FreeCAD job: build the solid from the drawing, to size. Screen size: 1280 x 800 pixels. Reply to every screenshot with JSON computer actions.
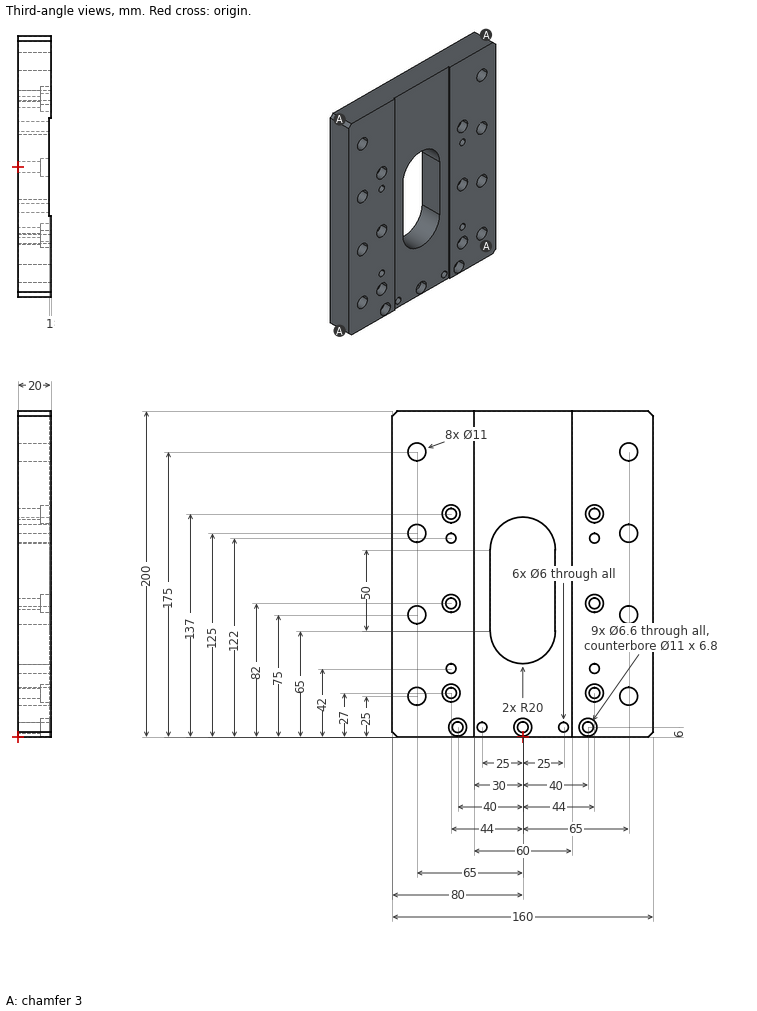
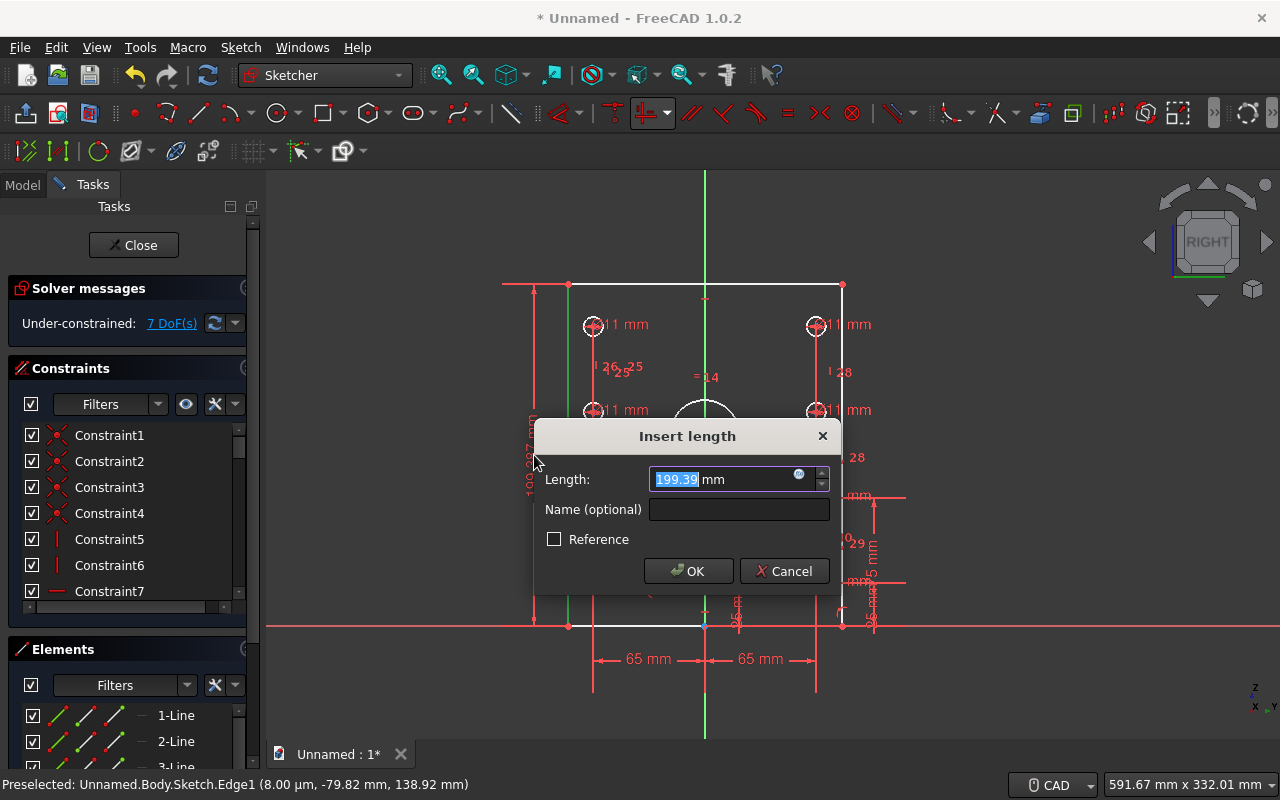
{"action": "type", "text": "200"}
{"action": "key", "text": "Return"}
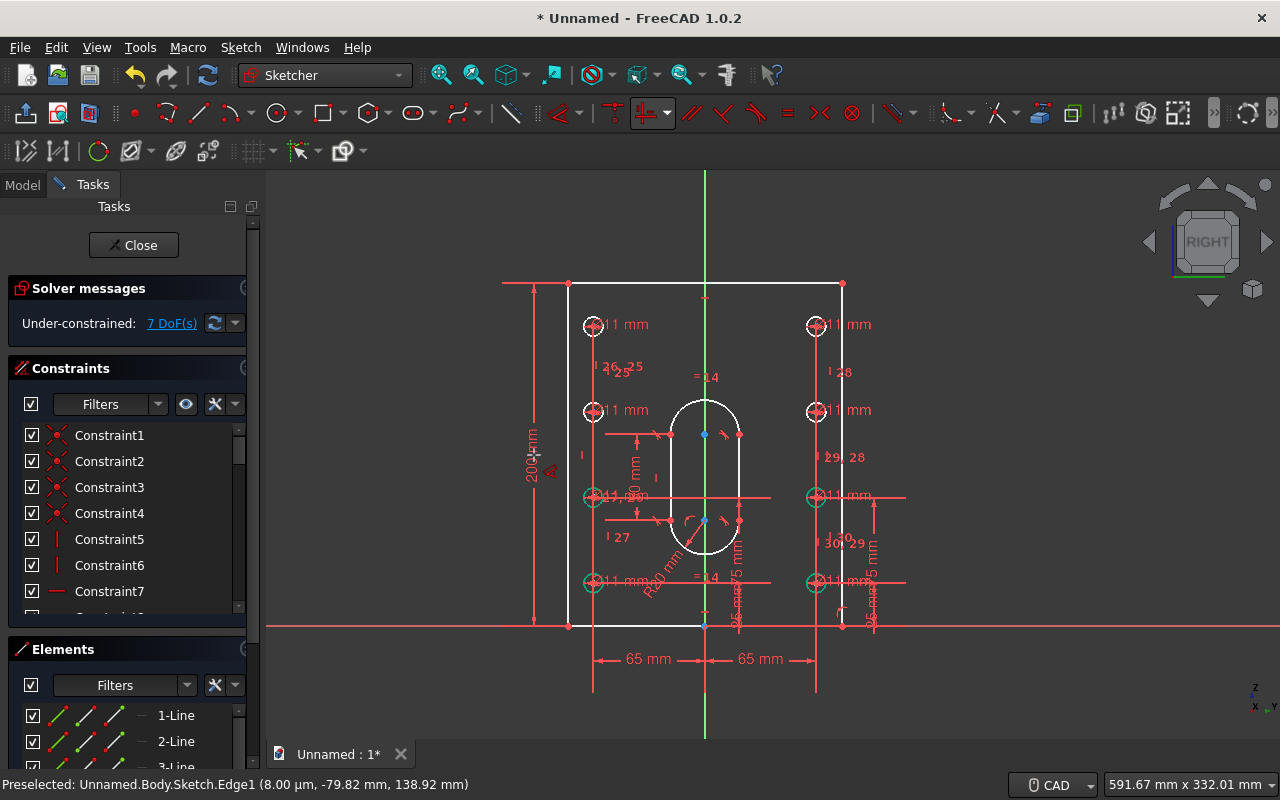
{"action": "left_click", "coordinate": [650, 626]}
{"action": "left_click", "coordinate": [642, 592]}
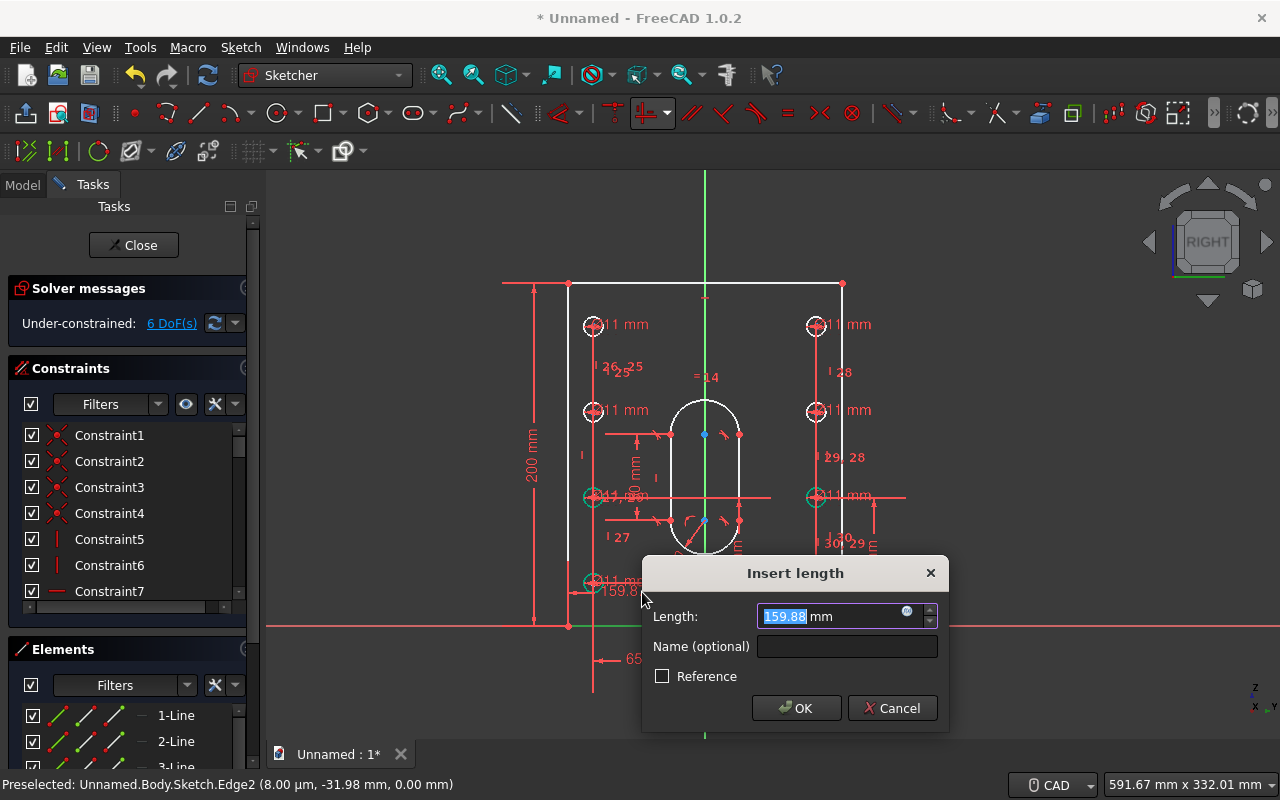
{"action": "type", "text": "160"}
{"action": "key", "text": "Return"}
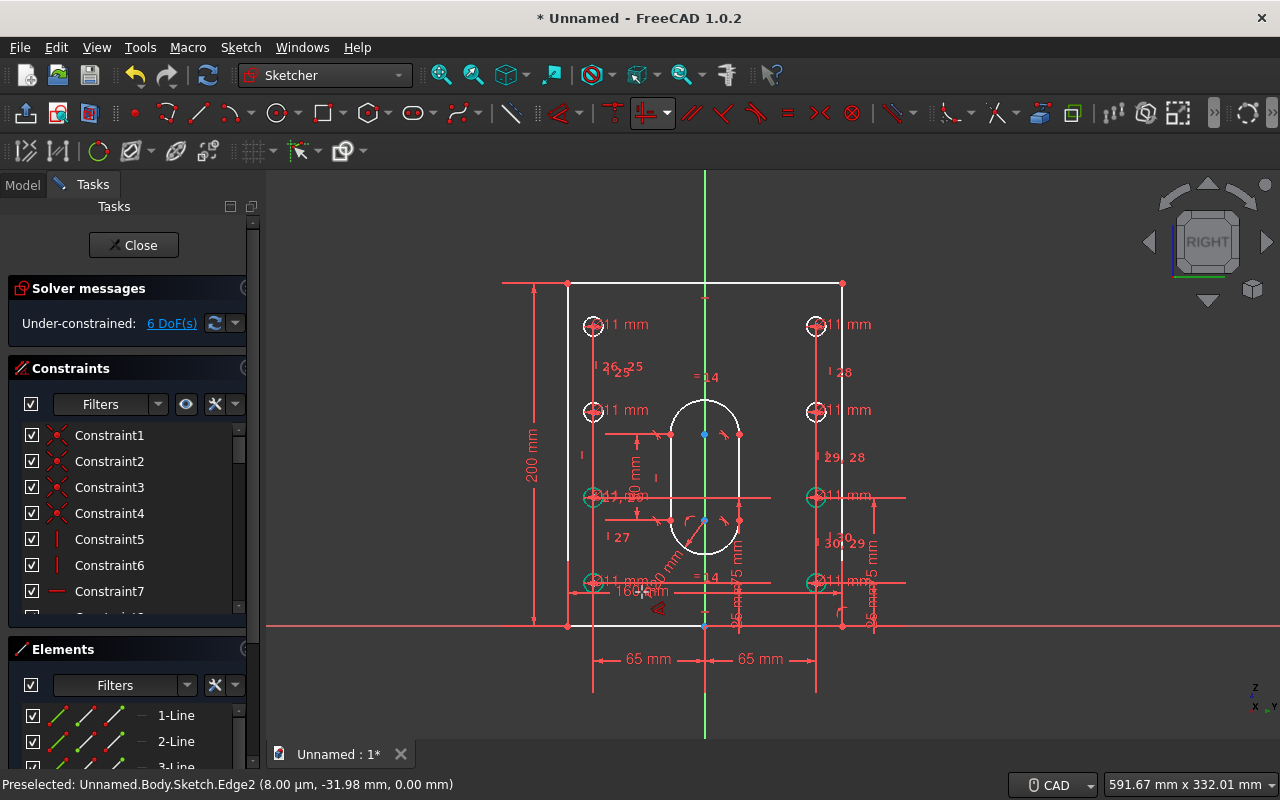
{"action": "left_click", "coordinate": [568, 283]}
{"action": "left_click", "coordinate": [636, 249]}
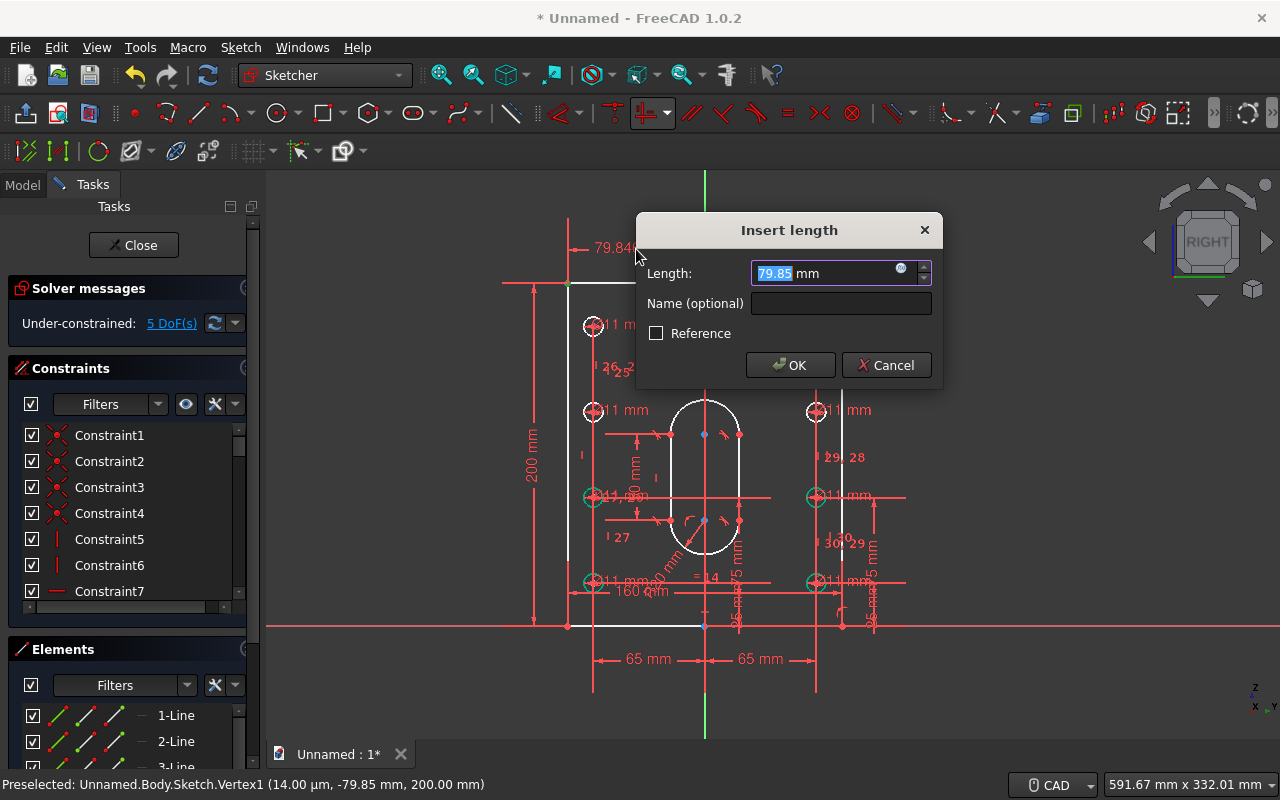
{"action": "type", "text": "80"}
{"action": "key", "text": "Return"}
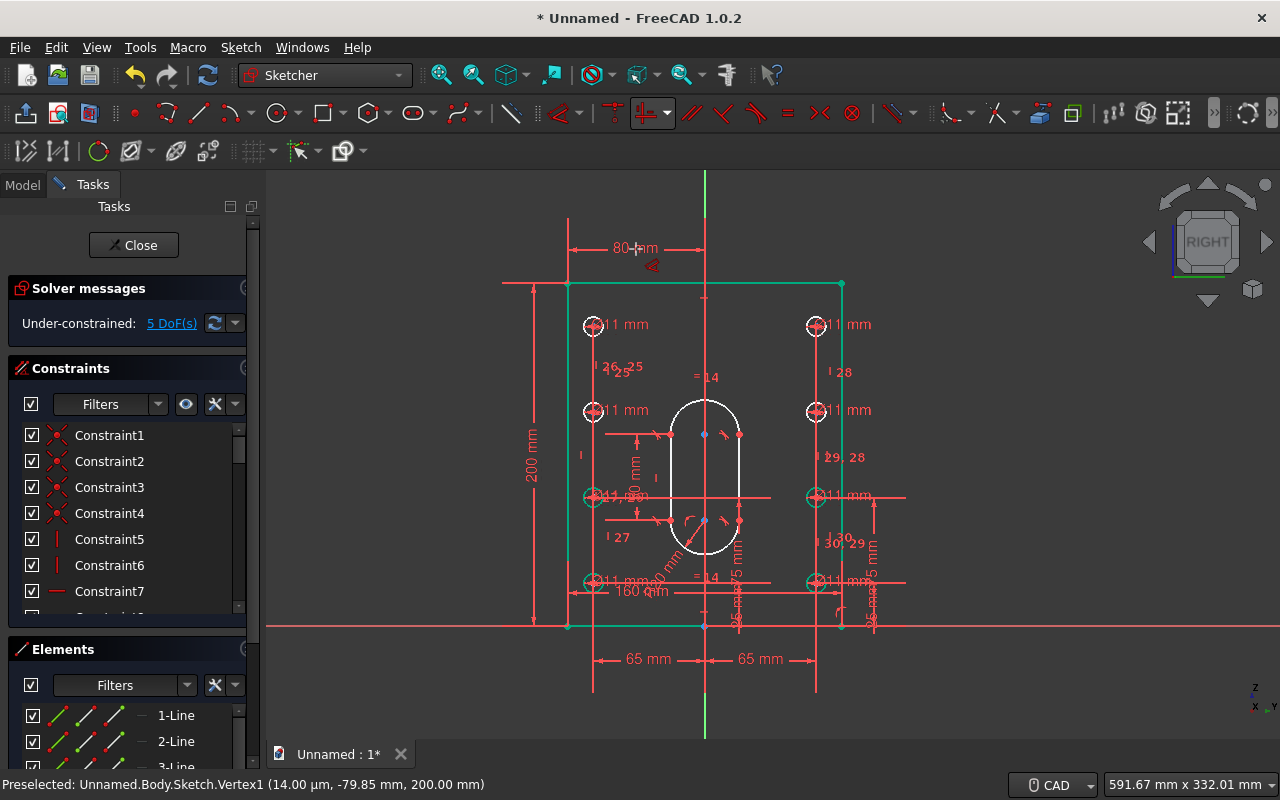
{"action": "left_click", "coordinate": [671, 520]}
{"action": "left_click", "coordinate": [637, 536]}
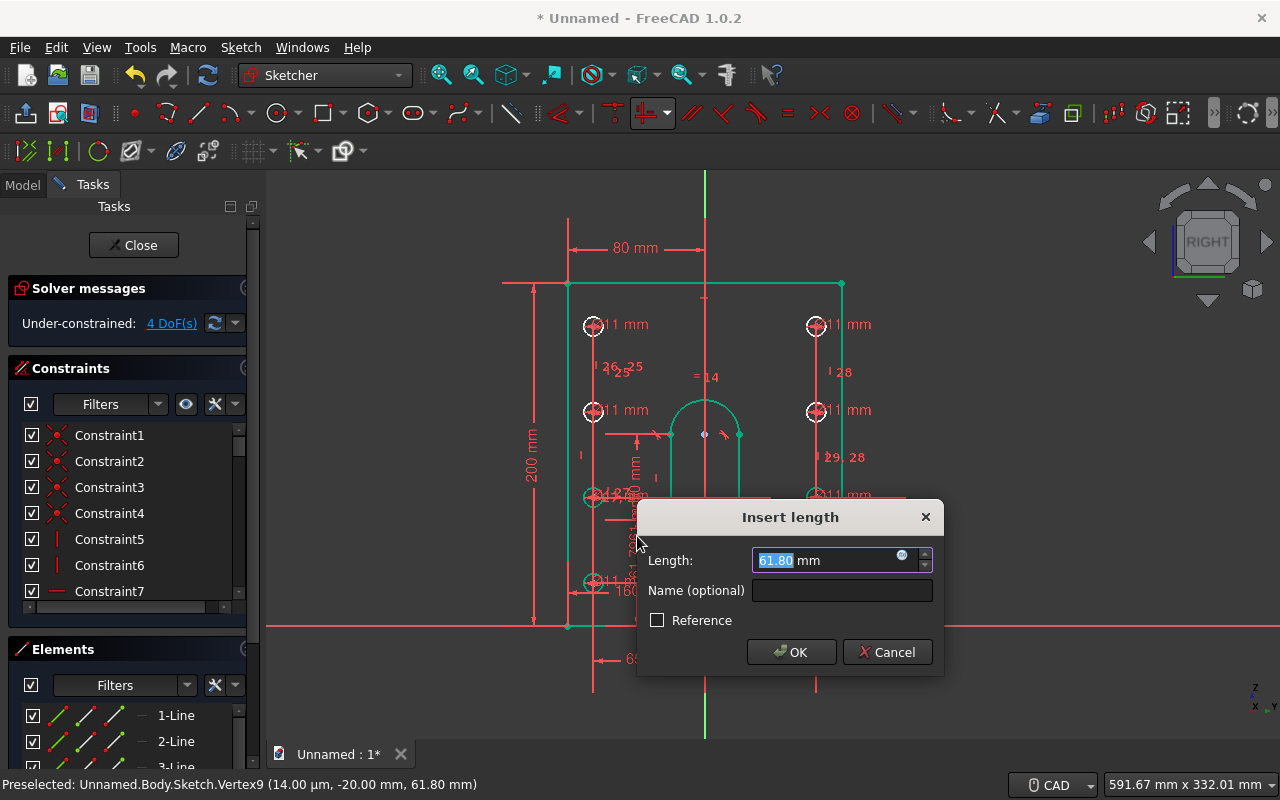
{"action": "type", "text": "65"}
{"action": "key", "text": "Return"}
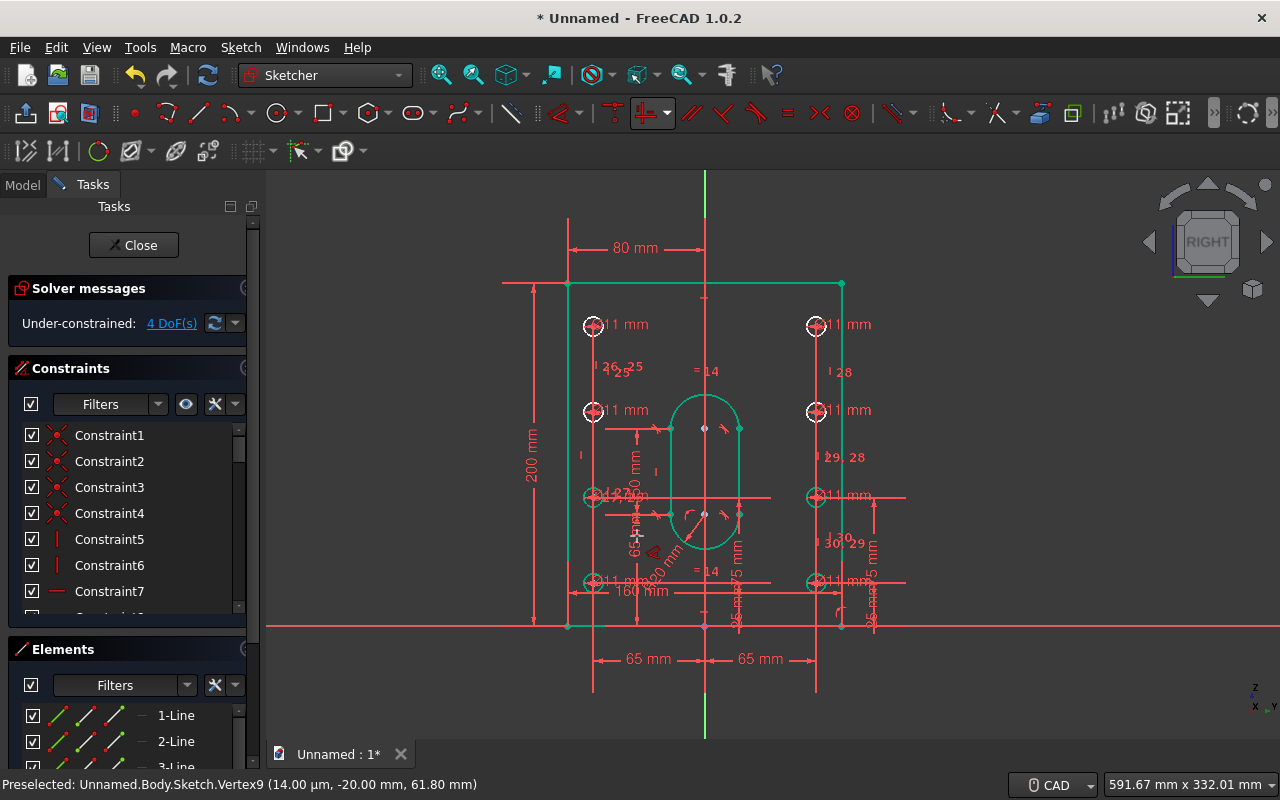
{"action": "left_click", "coordinate": [593, 327]}
{"action": "left_click", "coordinate": [739, 371]}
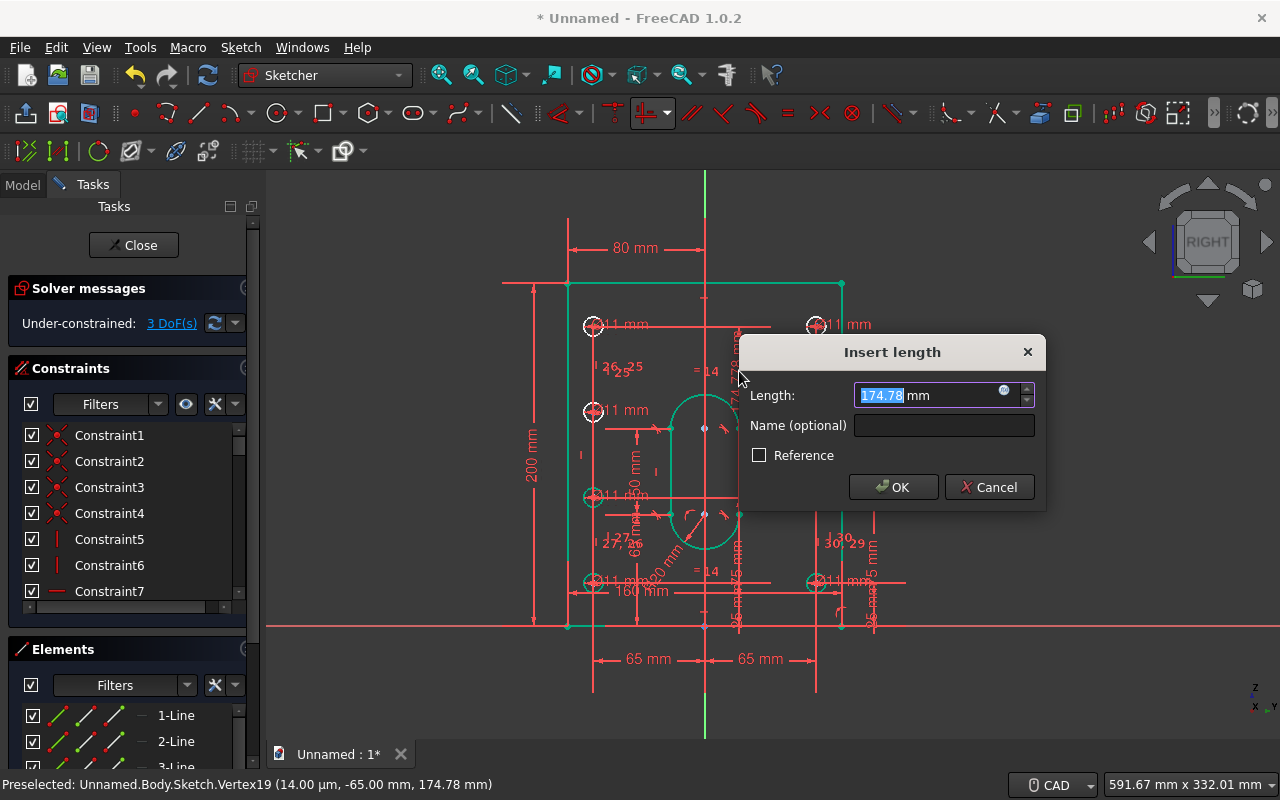
{"action": "type", "text": "175"}
{"action": "key", "text": "Return"}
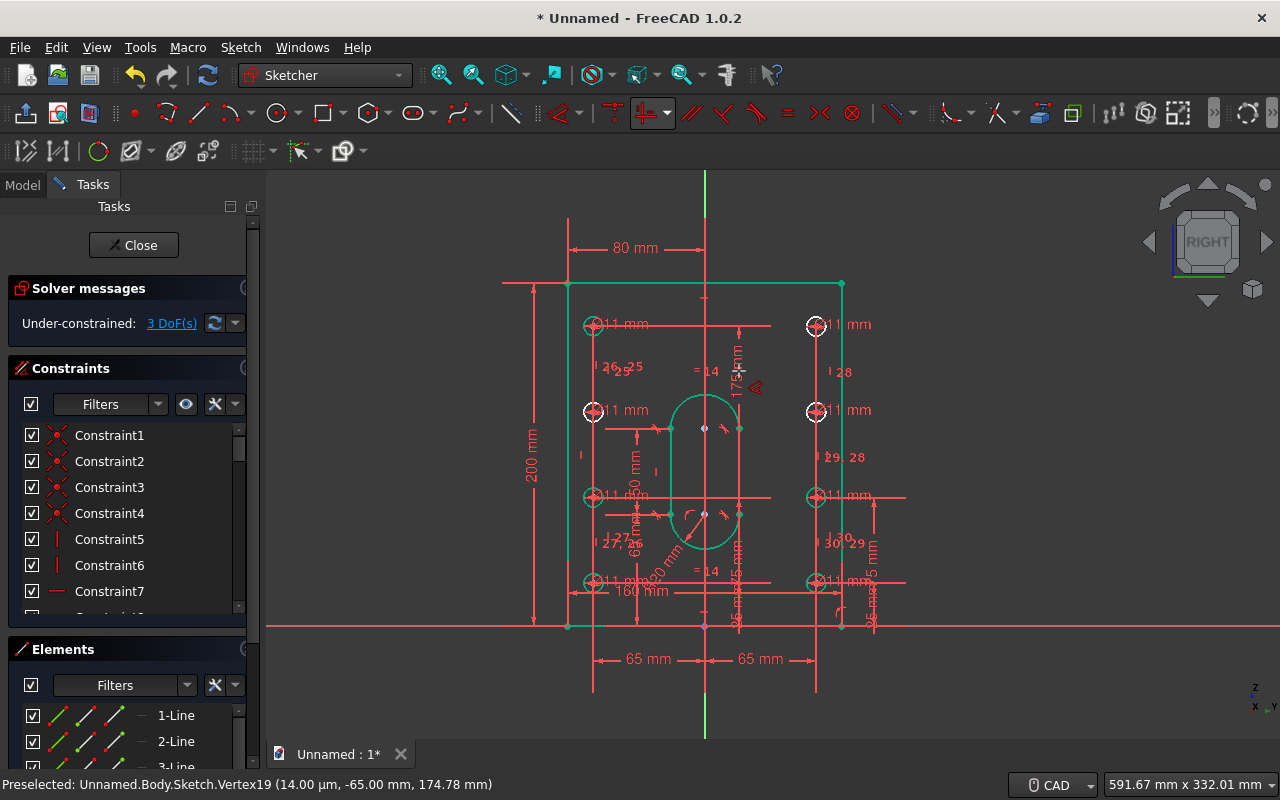
{"action": "left_click", "coordinate": [593, 412]}
{"action": "left_click", "coordinate": [535, 519]}